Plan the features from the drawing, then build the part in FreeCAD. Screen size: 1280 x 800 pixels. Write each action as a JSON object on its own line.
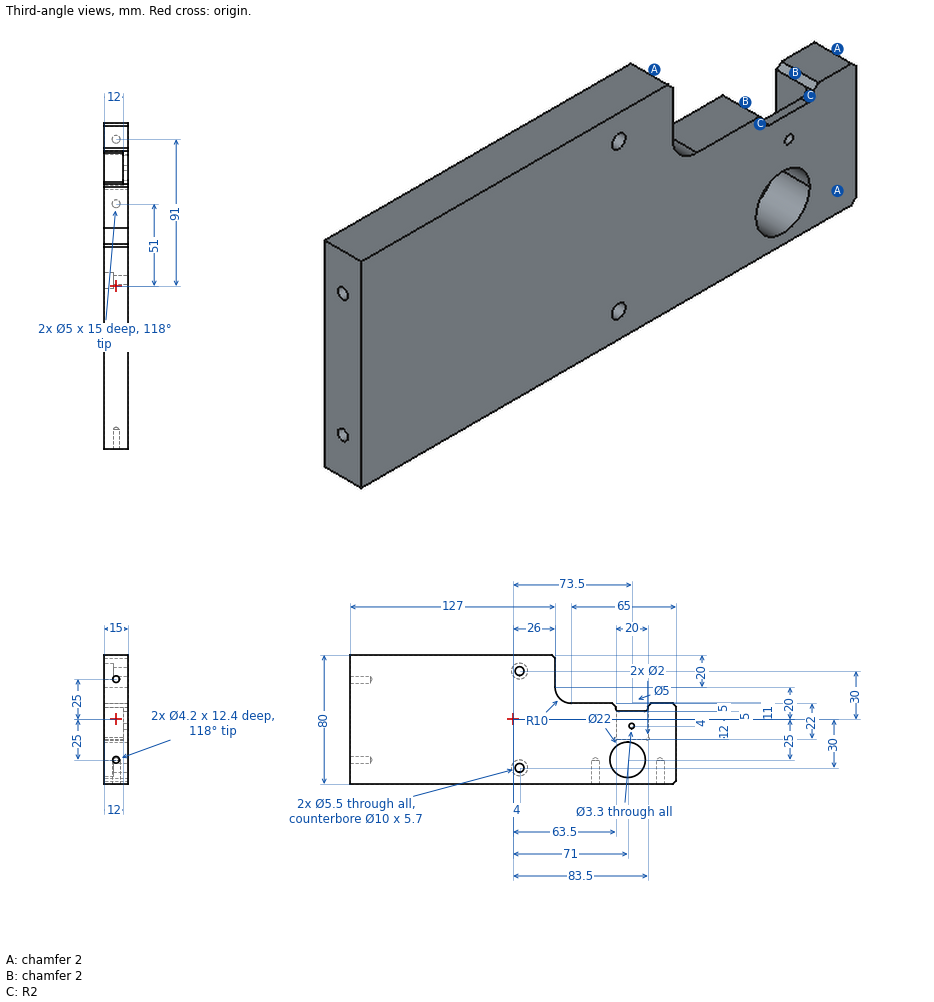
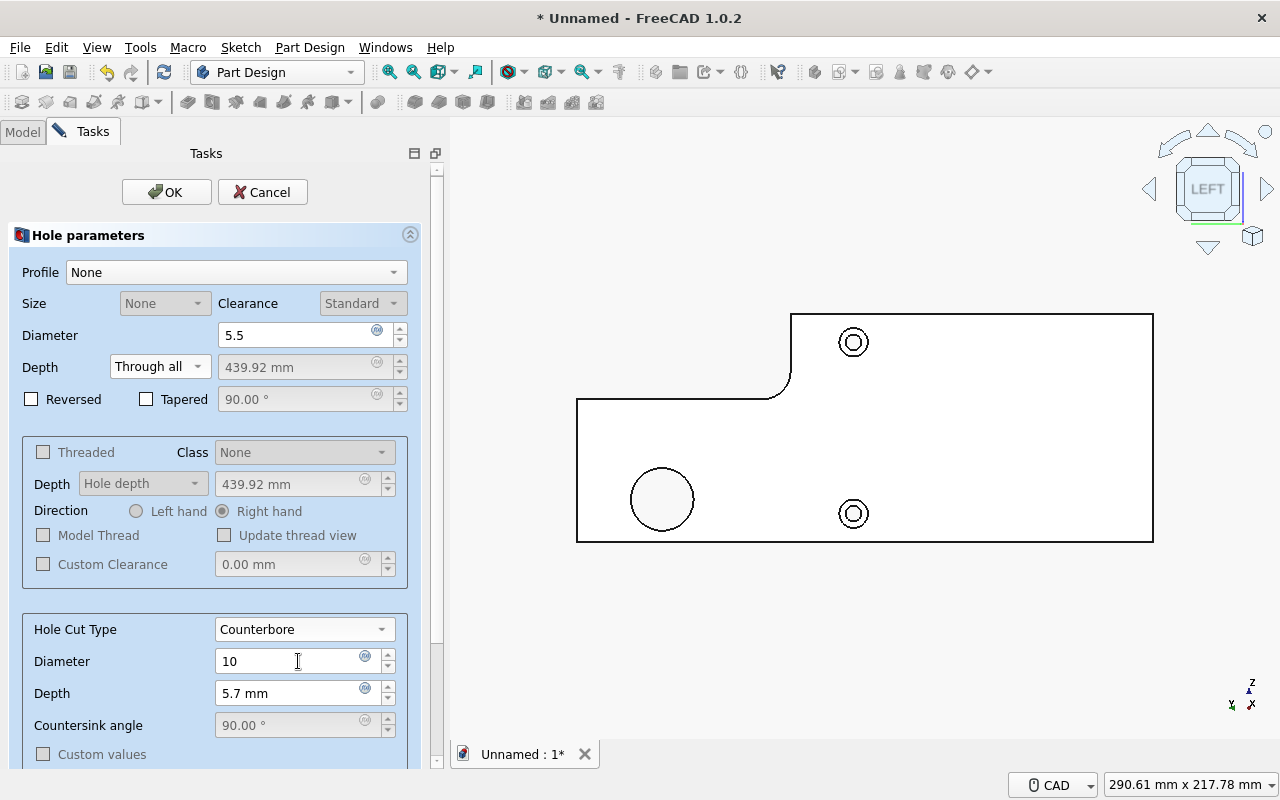
{"action": "left_click", "coordinate": [167, 192]}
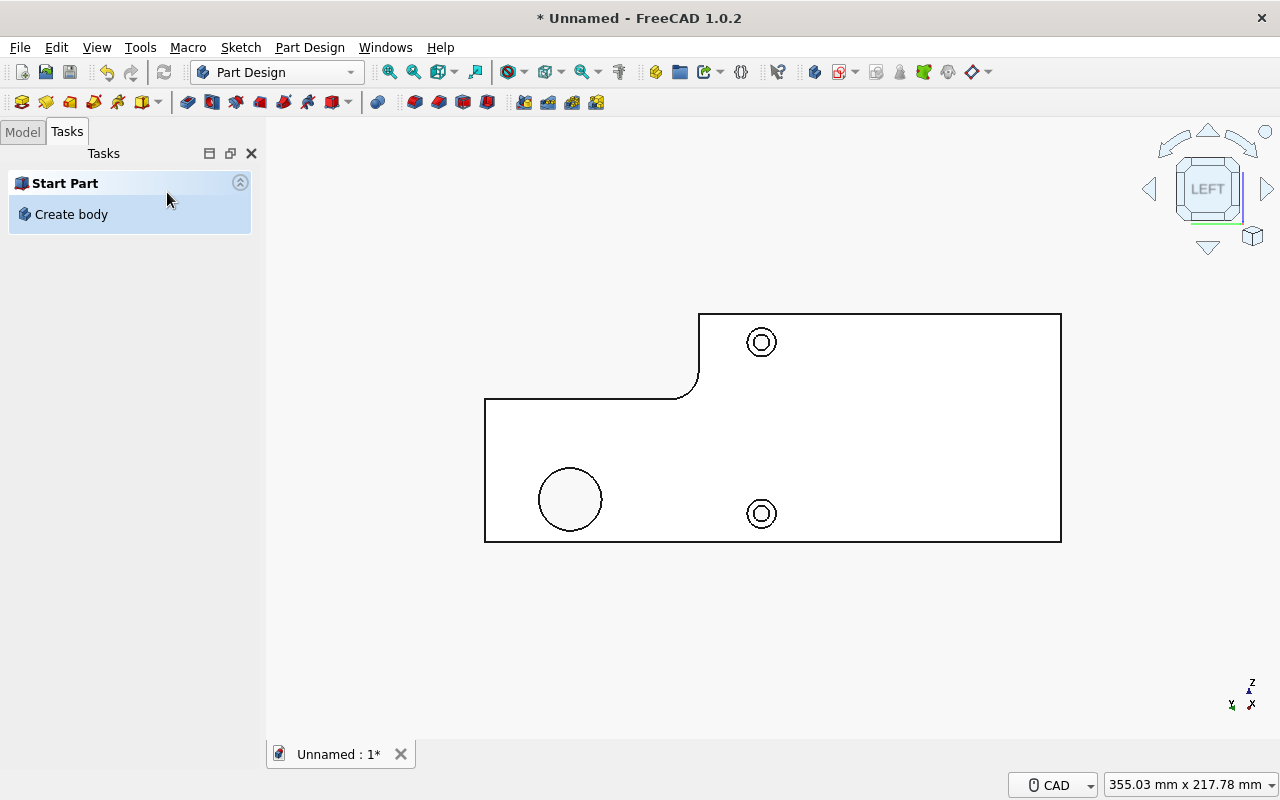
{"action": "key", "text": "5"}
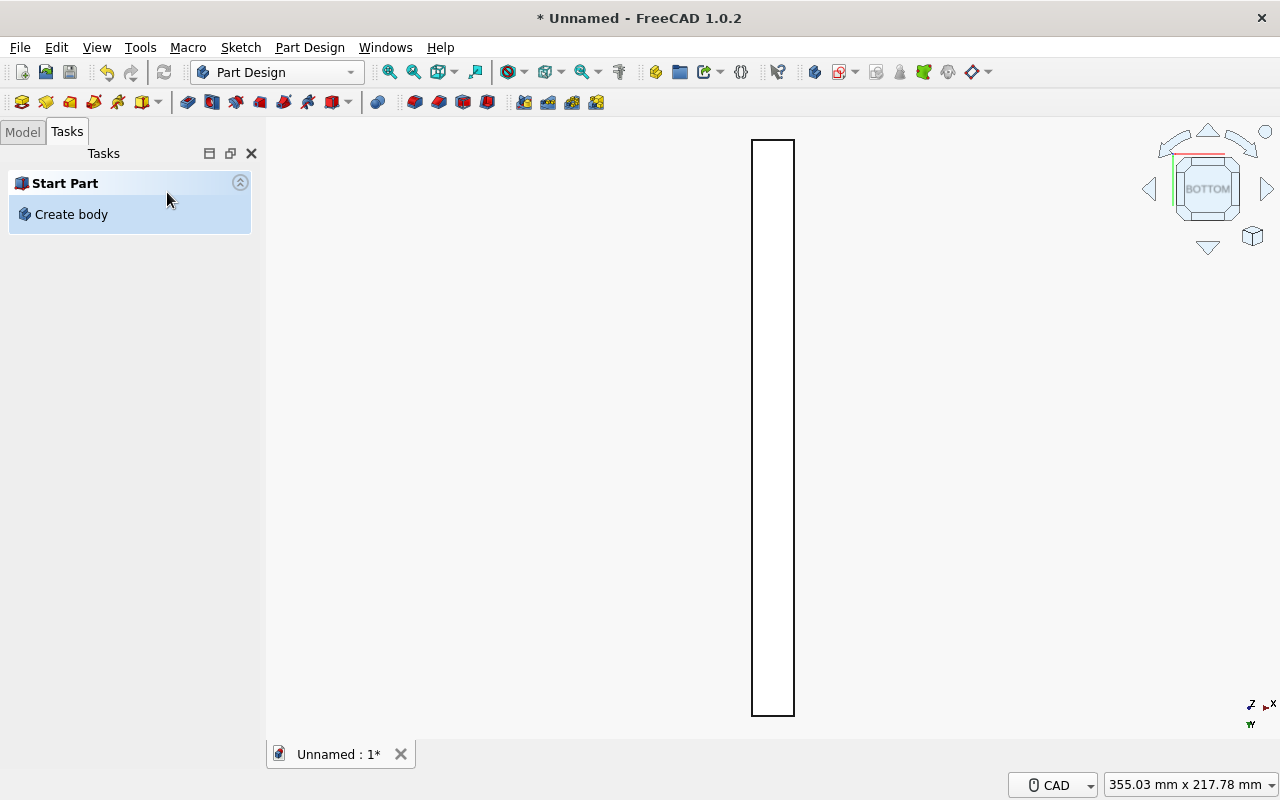
{"action": "left_click", "coordinate": [773, 674]}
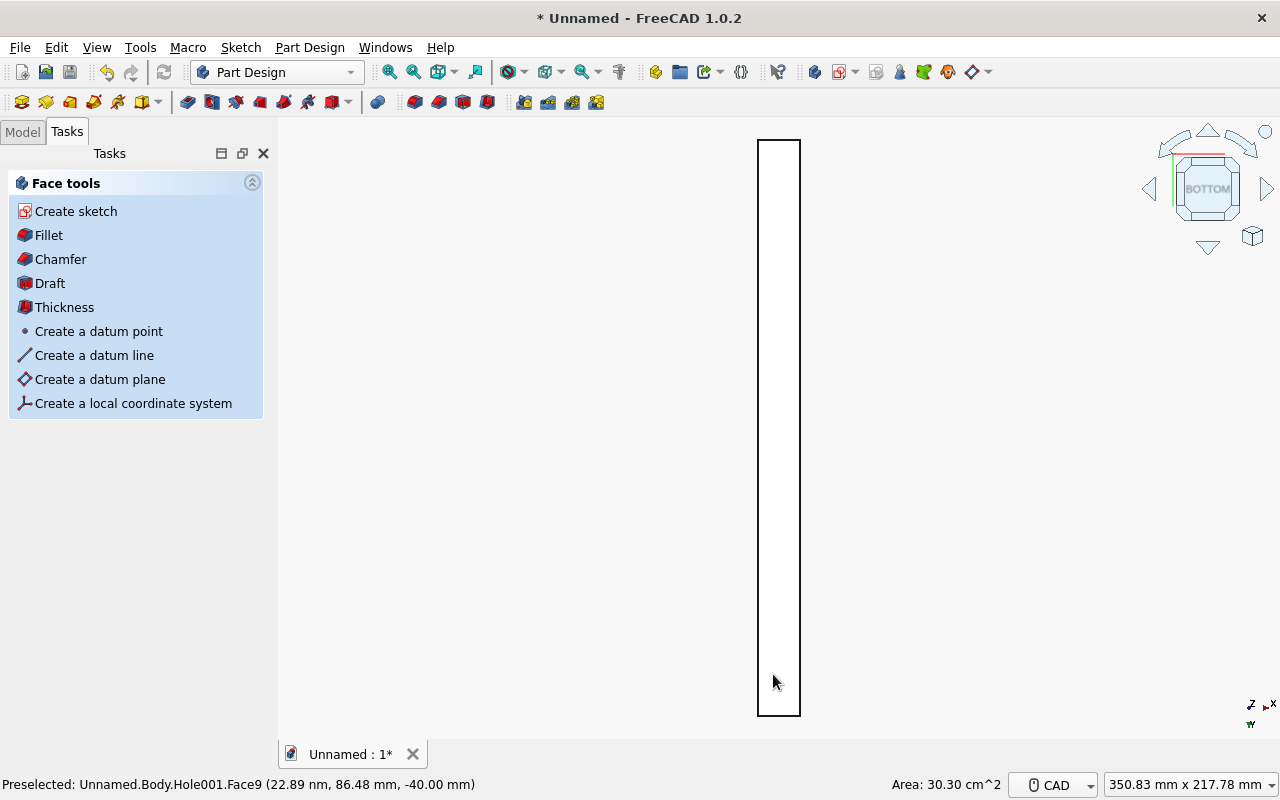
{"action": "left_click", "coordinate": [840, 72]}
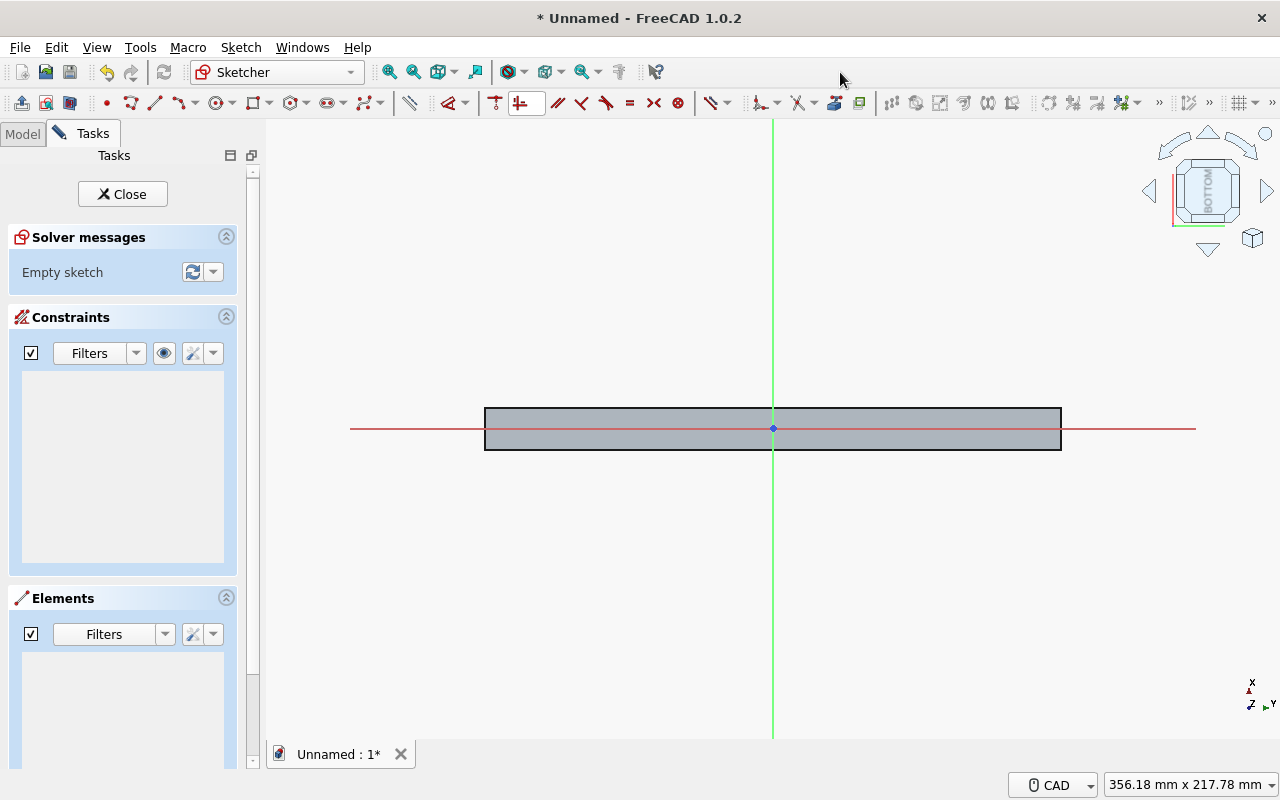
{"action": "scroll", "coordinate": [1071, 429], "scroll_direction": "up", "scroll_amount": 4}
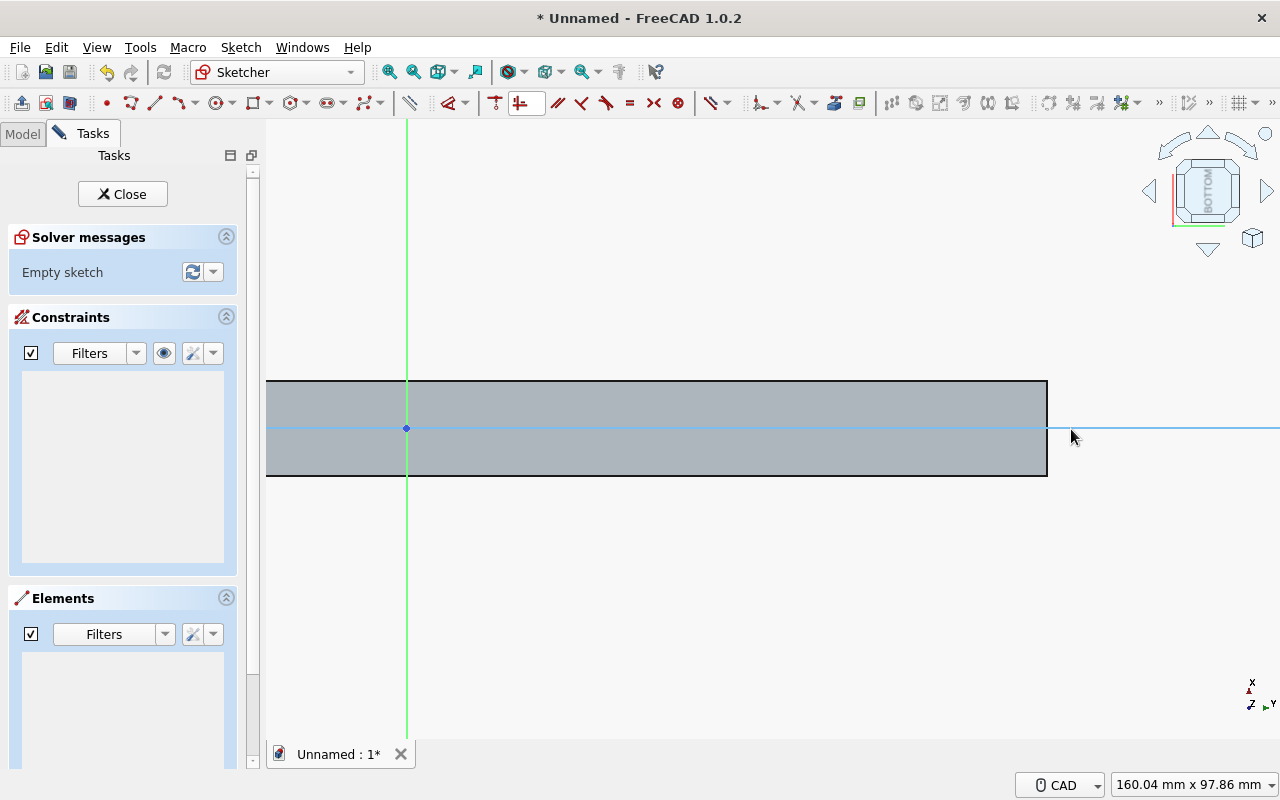
{"action": "left_click", "coordinate": [216, 104]}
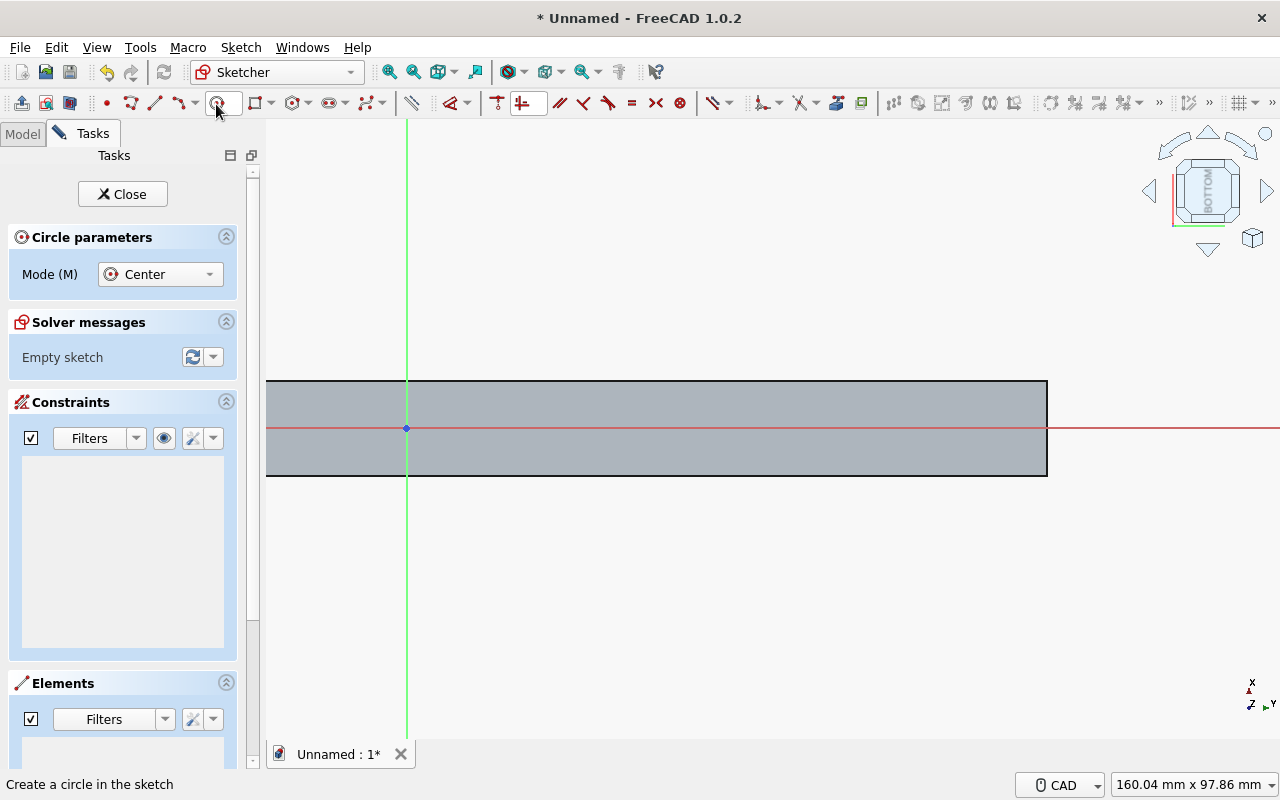
{"action": "scroll", "coordinate": [730, 428], "scroll_direction": "up", "scroll_amount": 2}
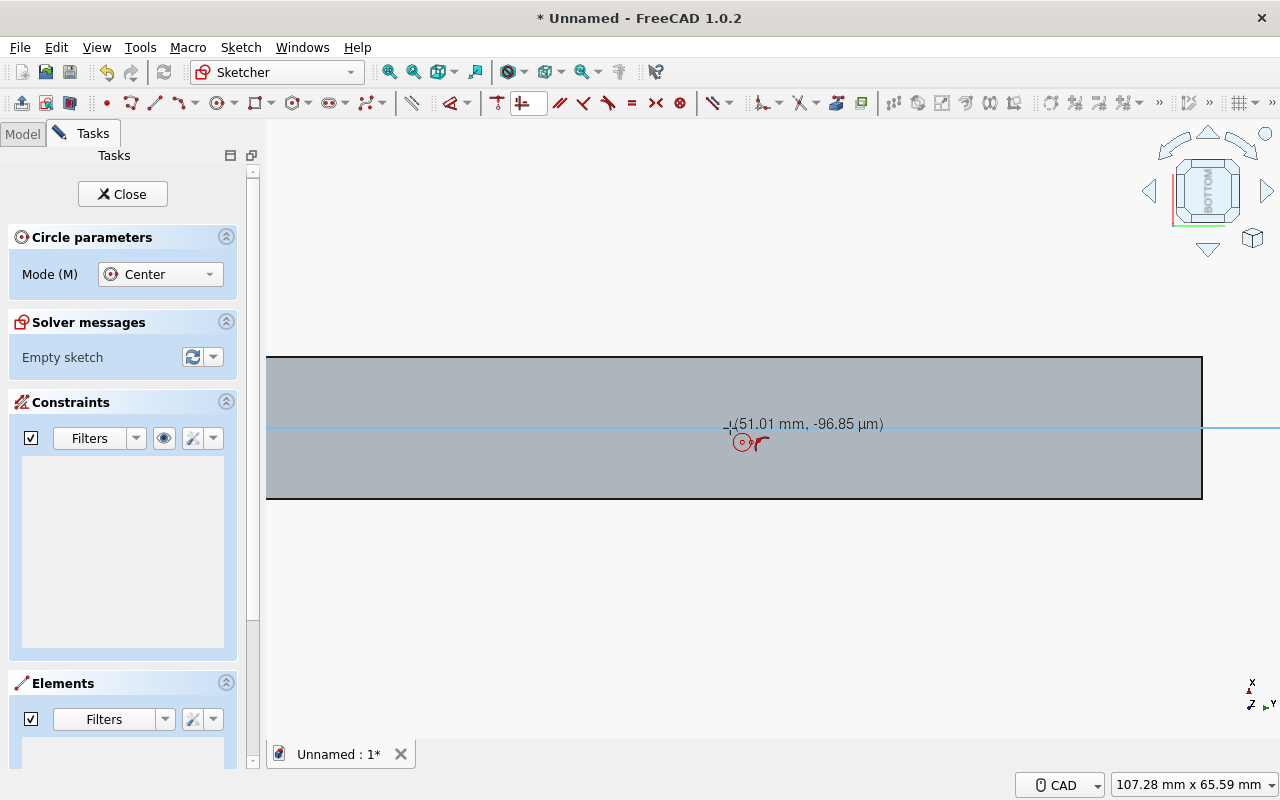
{"action": "left_click", "coordinate": [730, 428]}
{"action": "left_click", "coordinate": [746, 412]}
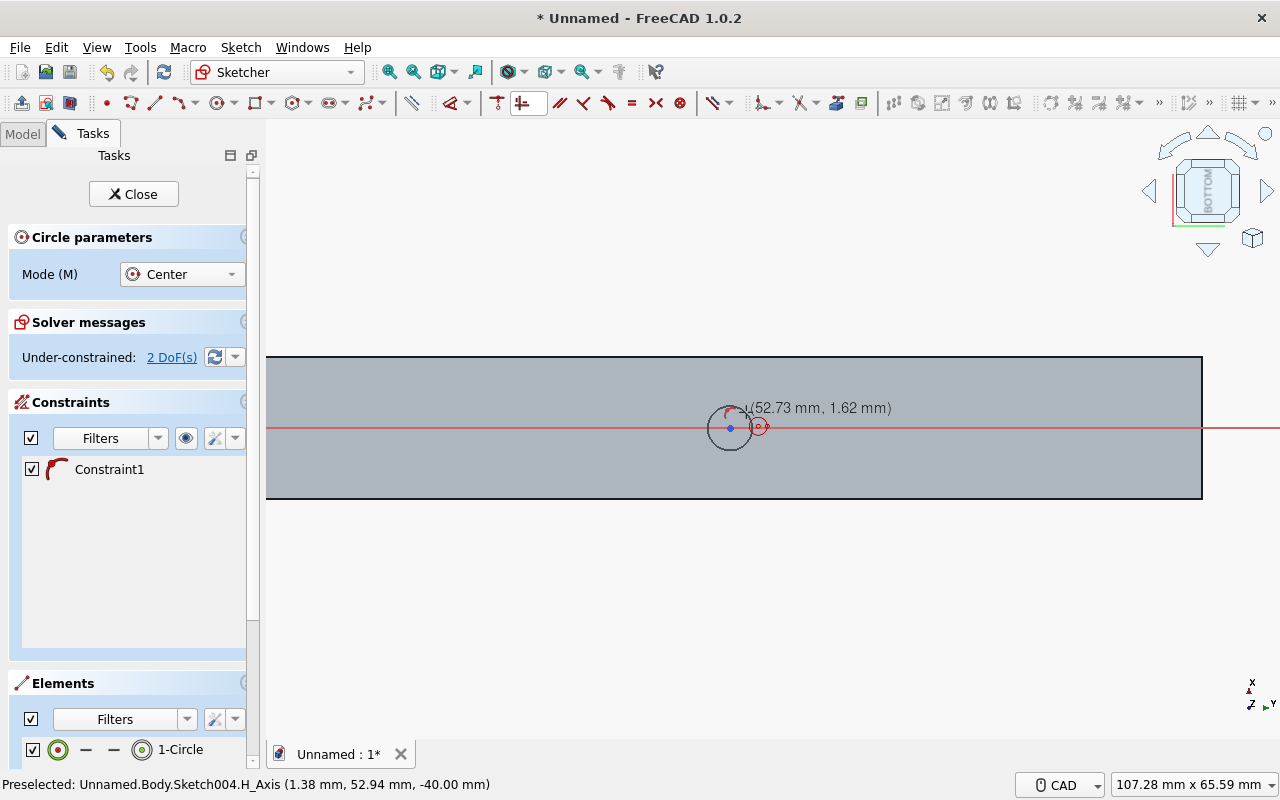
{"action": "left_click", "coordinate": [1108, 428]}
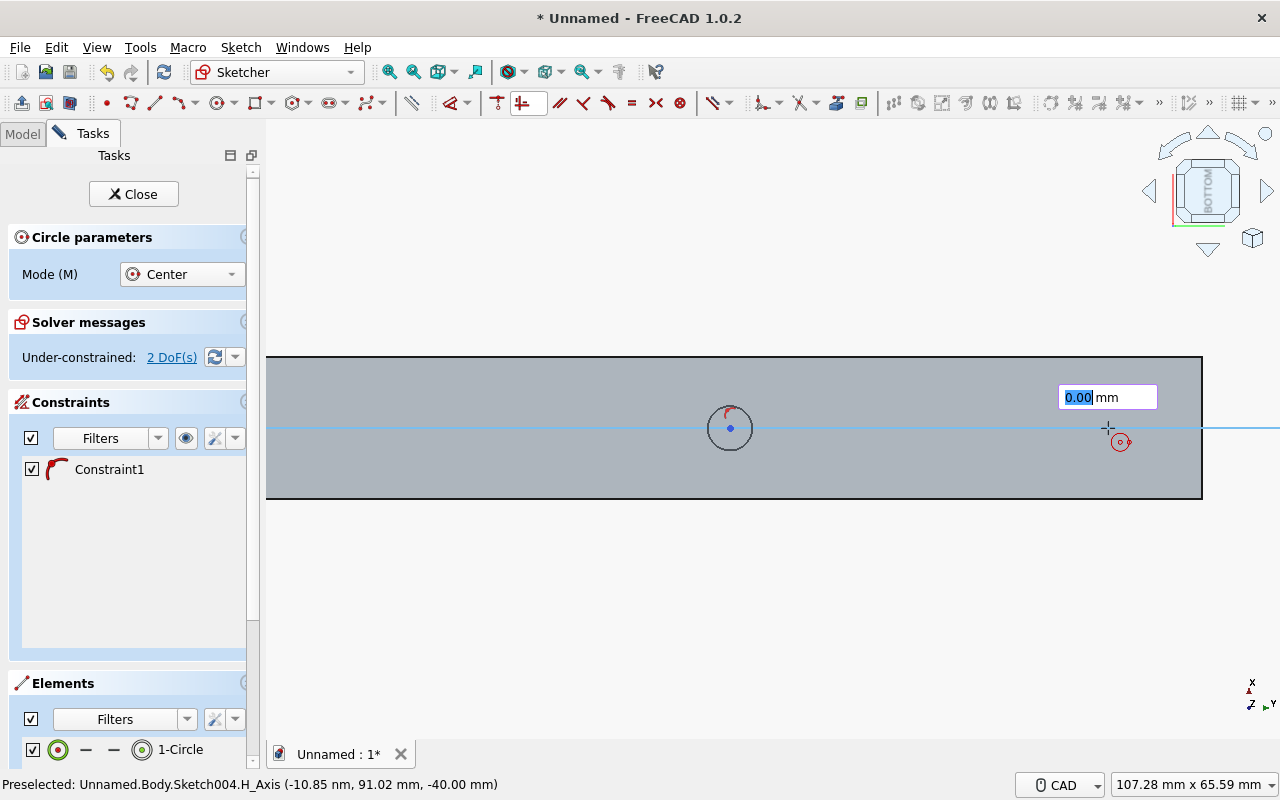
{"action": "scroll", "coordinate": [735, 430], "scroll_direction": "down", "scroll_amount": 2}